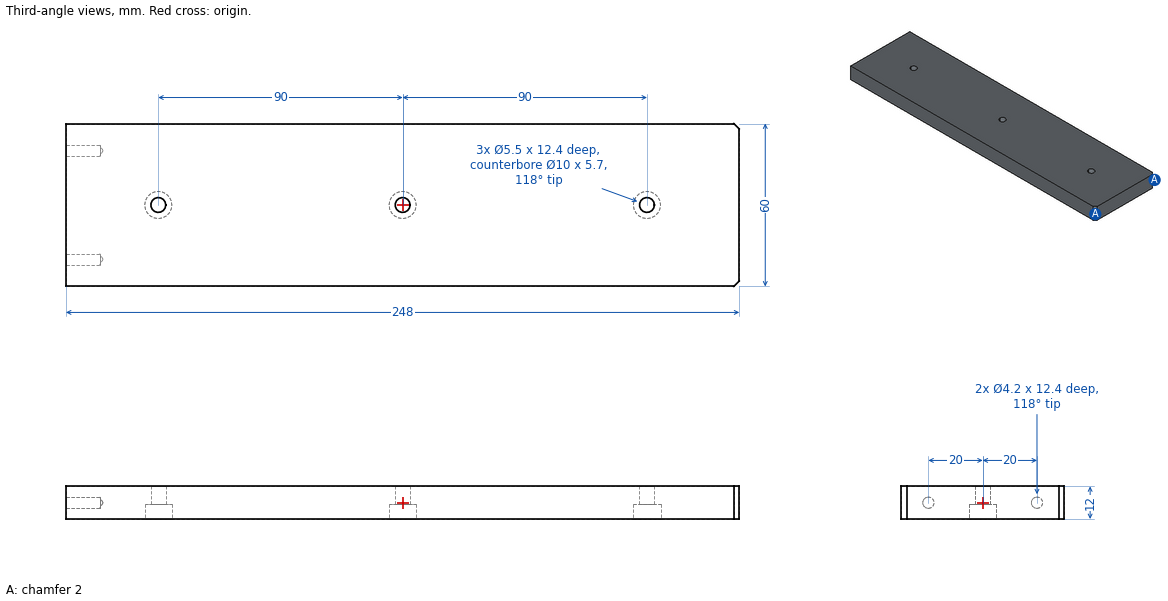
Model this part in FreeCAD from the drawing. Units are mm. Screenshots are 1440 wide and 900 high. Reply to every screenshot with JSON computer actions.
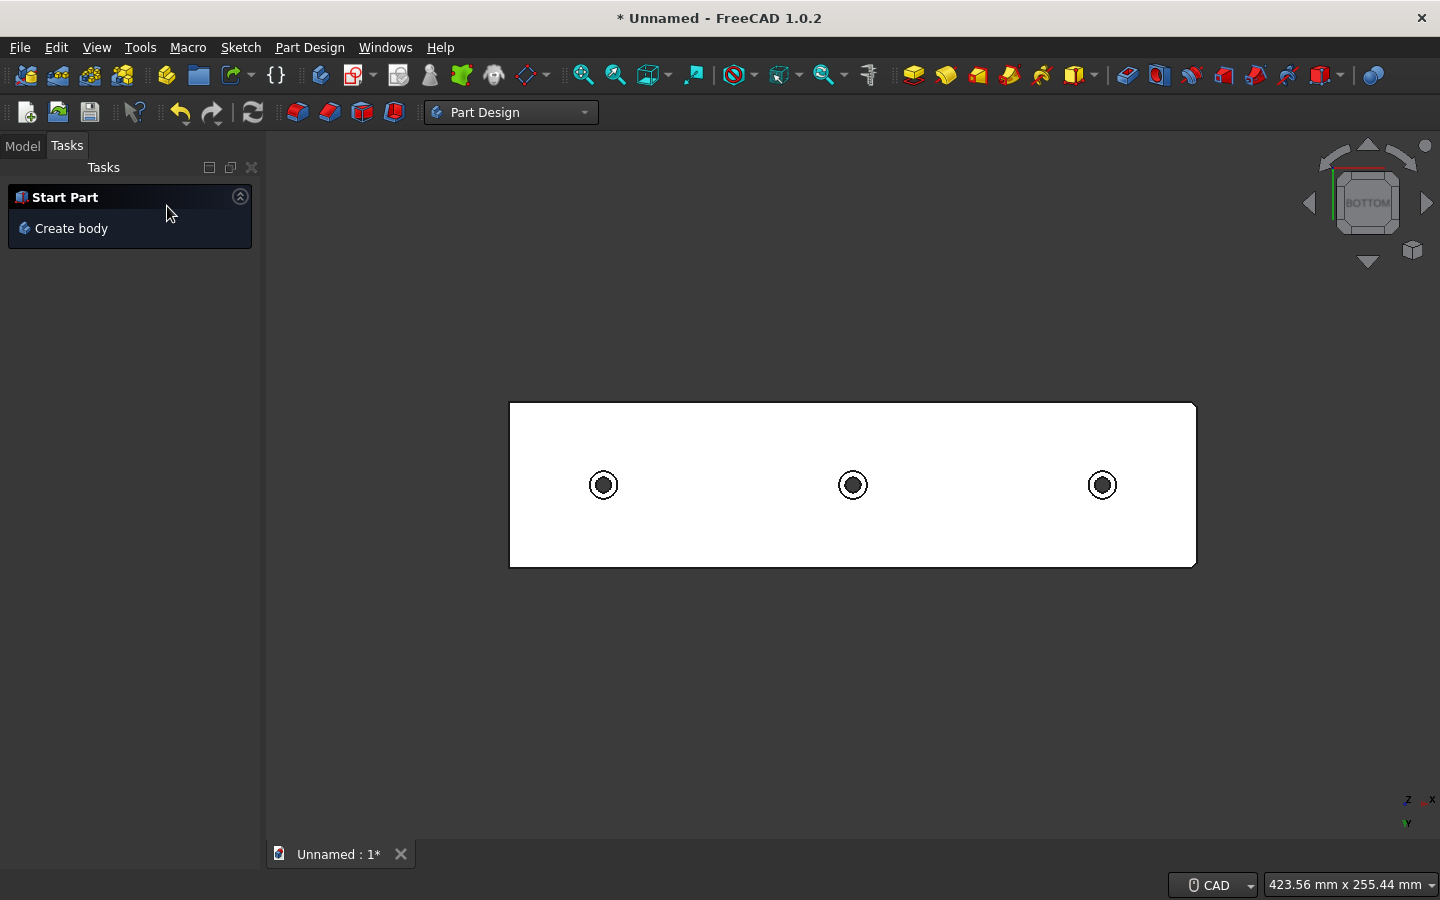
{"action": "key", "text": "0"}